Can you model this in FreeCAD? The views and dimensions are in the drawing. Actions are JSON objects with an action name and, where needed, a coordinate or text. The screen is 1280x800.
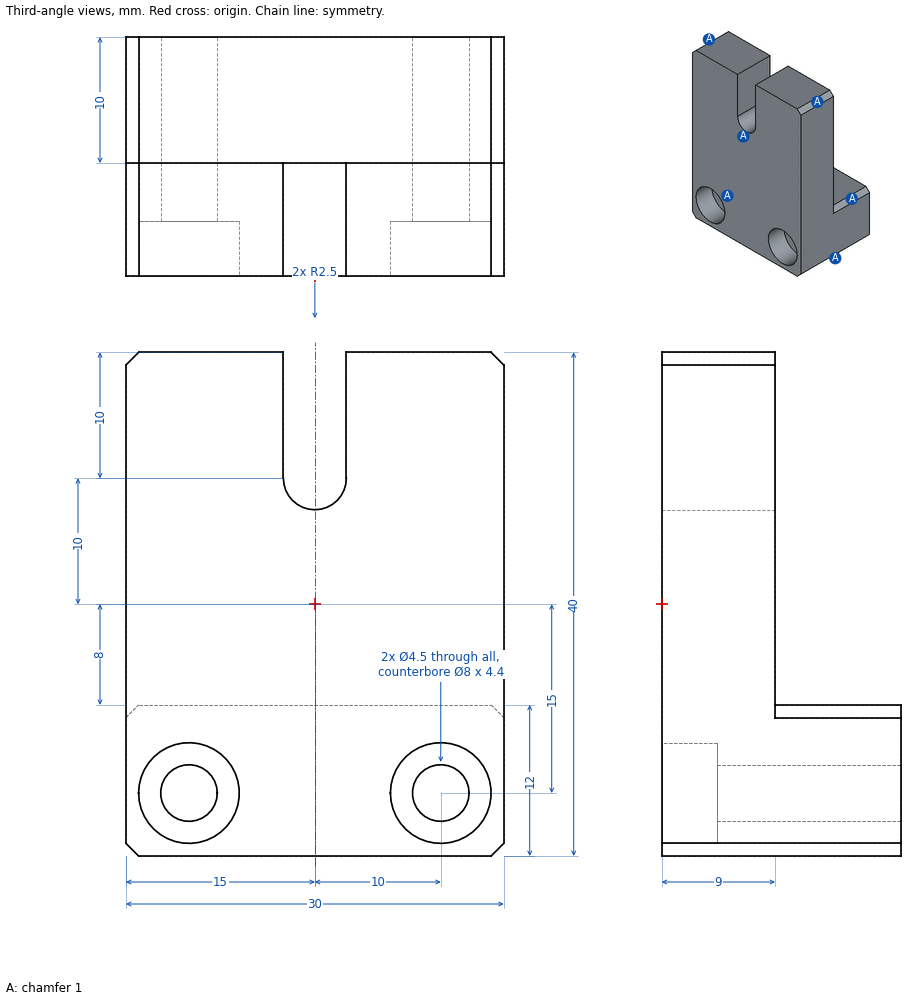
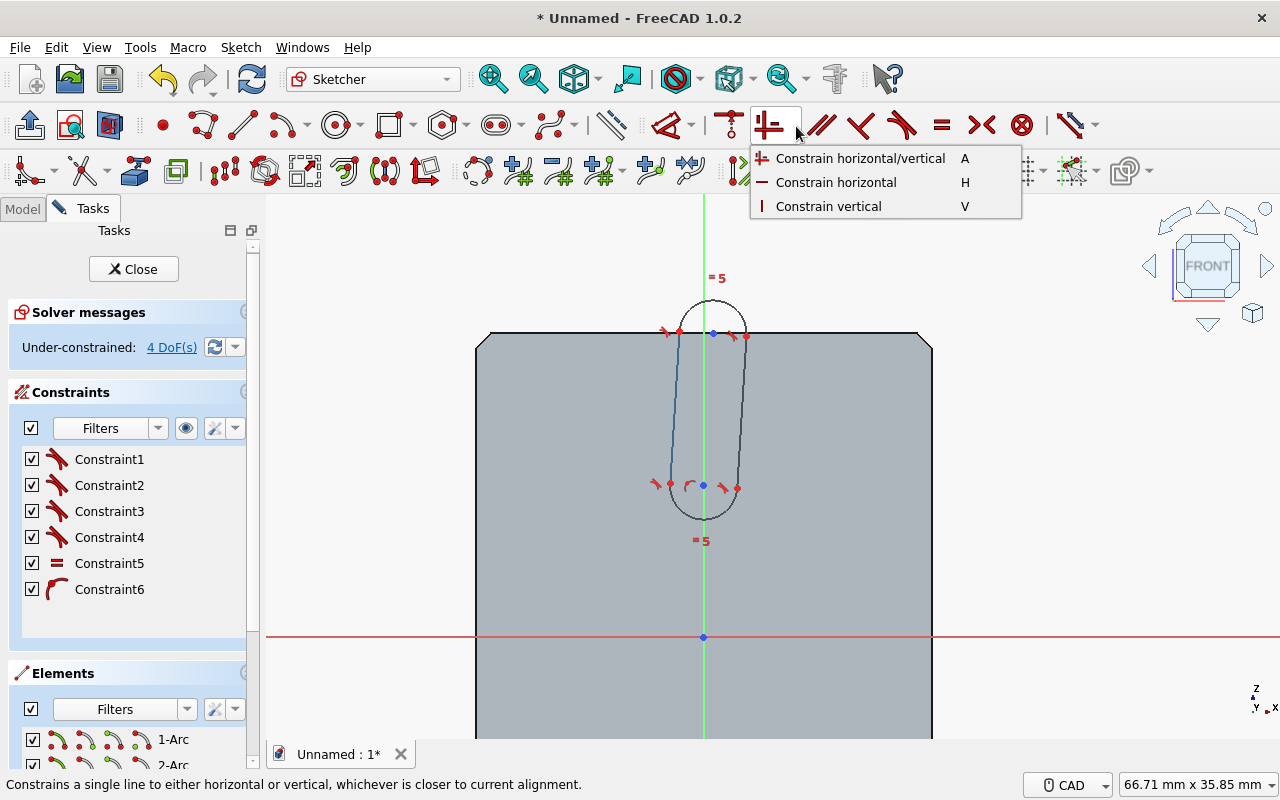
{"action": "left_click", "coordinate": [886, 206]}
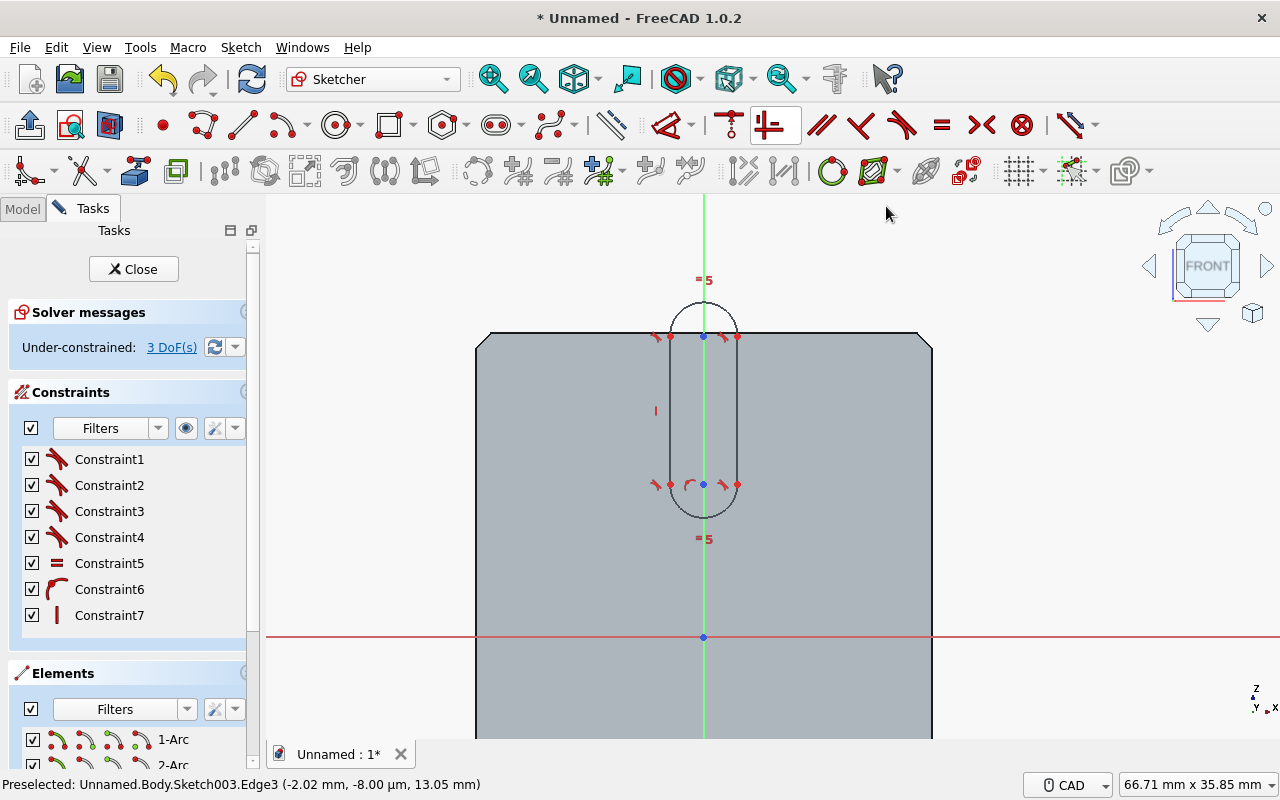
{"action": "left_click", "coordinate": [666, 126]}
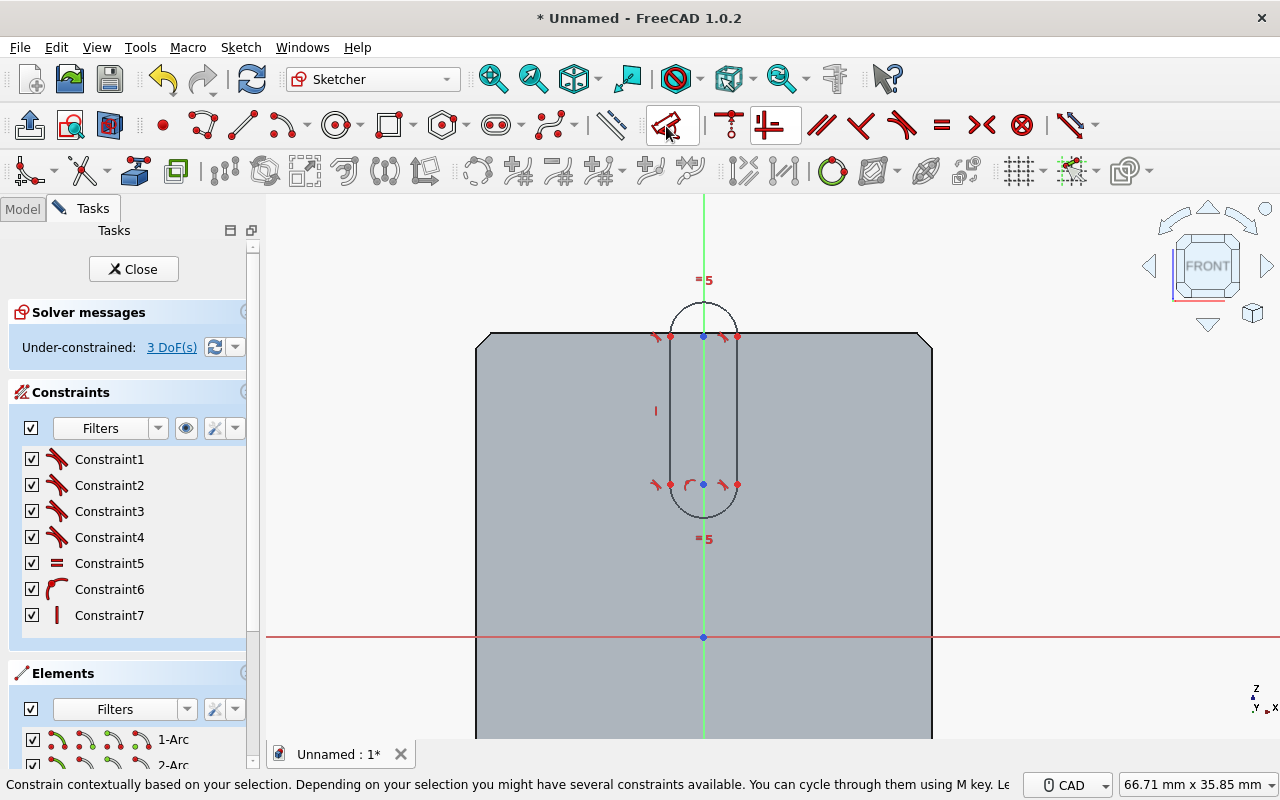
{"action": "left_click", "coordinate": [684, 511]}
{"action": "left_click", "coordinate": [665, 537]}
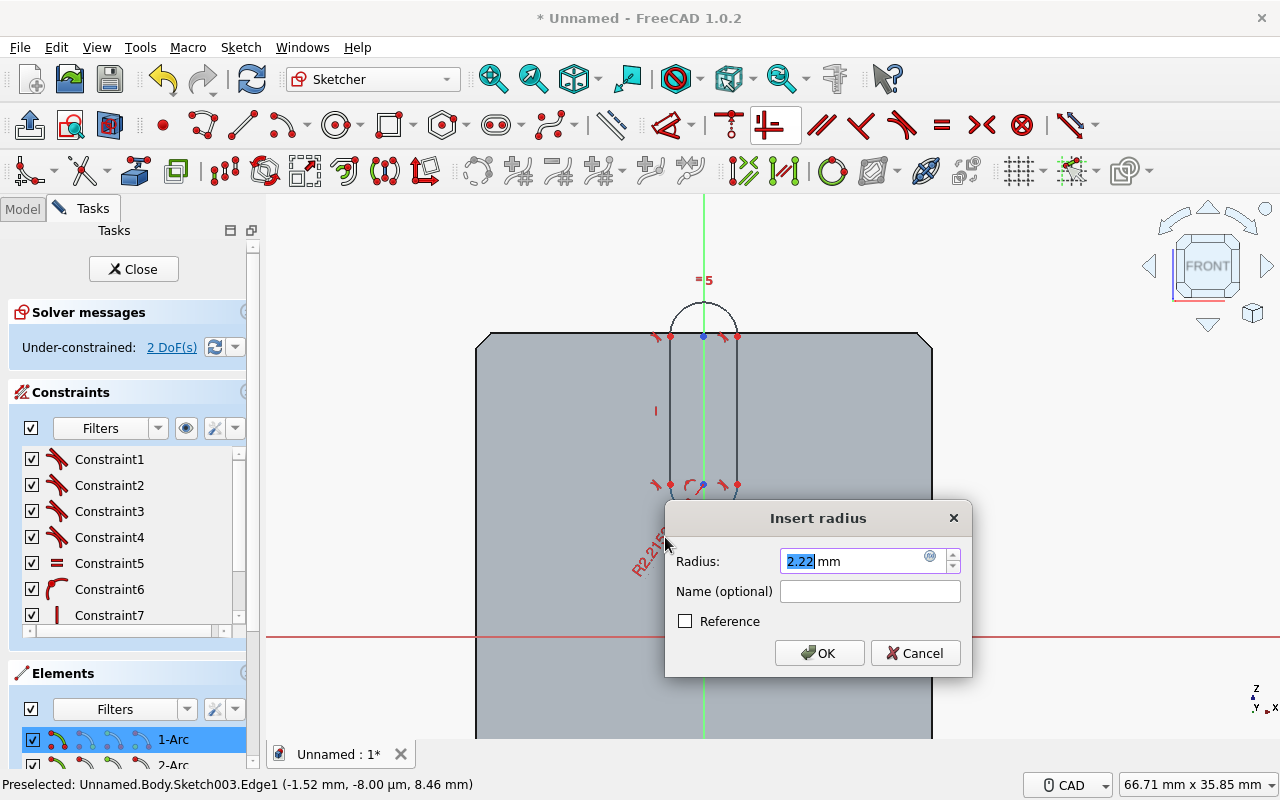
{"action": "type", "text": "2.5"}
{"action": "key", "text": "Return"}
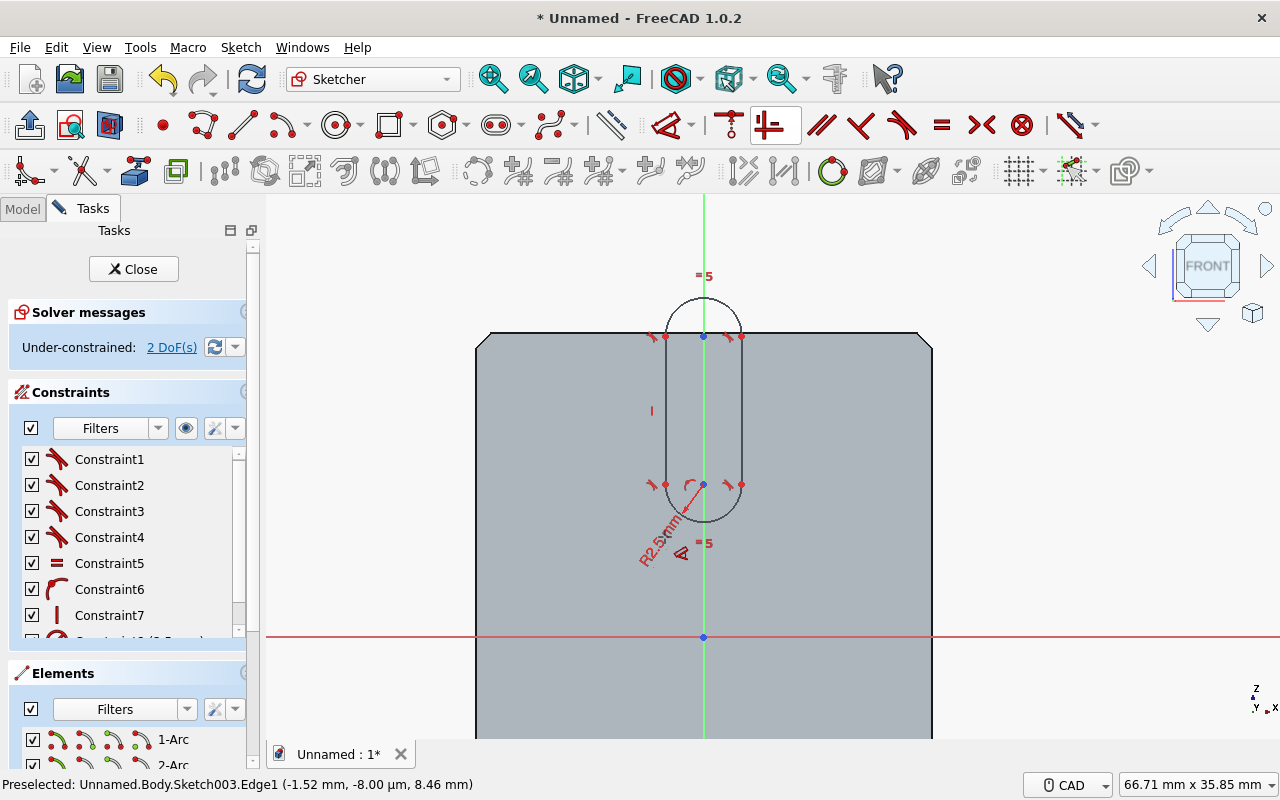
{"action": "left_click", "coordinate": [666, 440]}
{"action": "left_click", "coordinate": [632, 410]}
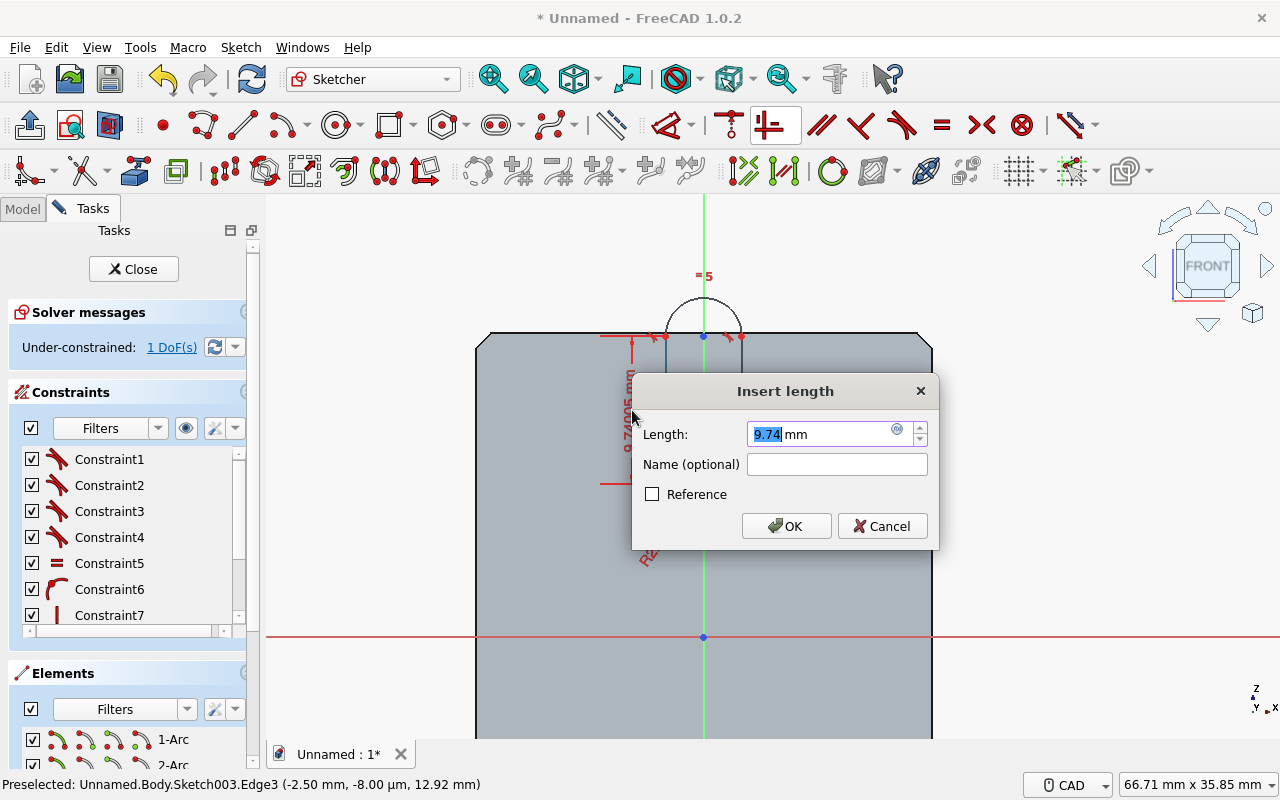
{"action": "type", "text": "10"}
{"action": "key", "text": "Return"}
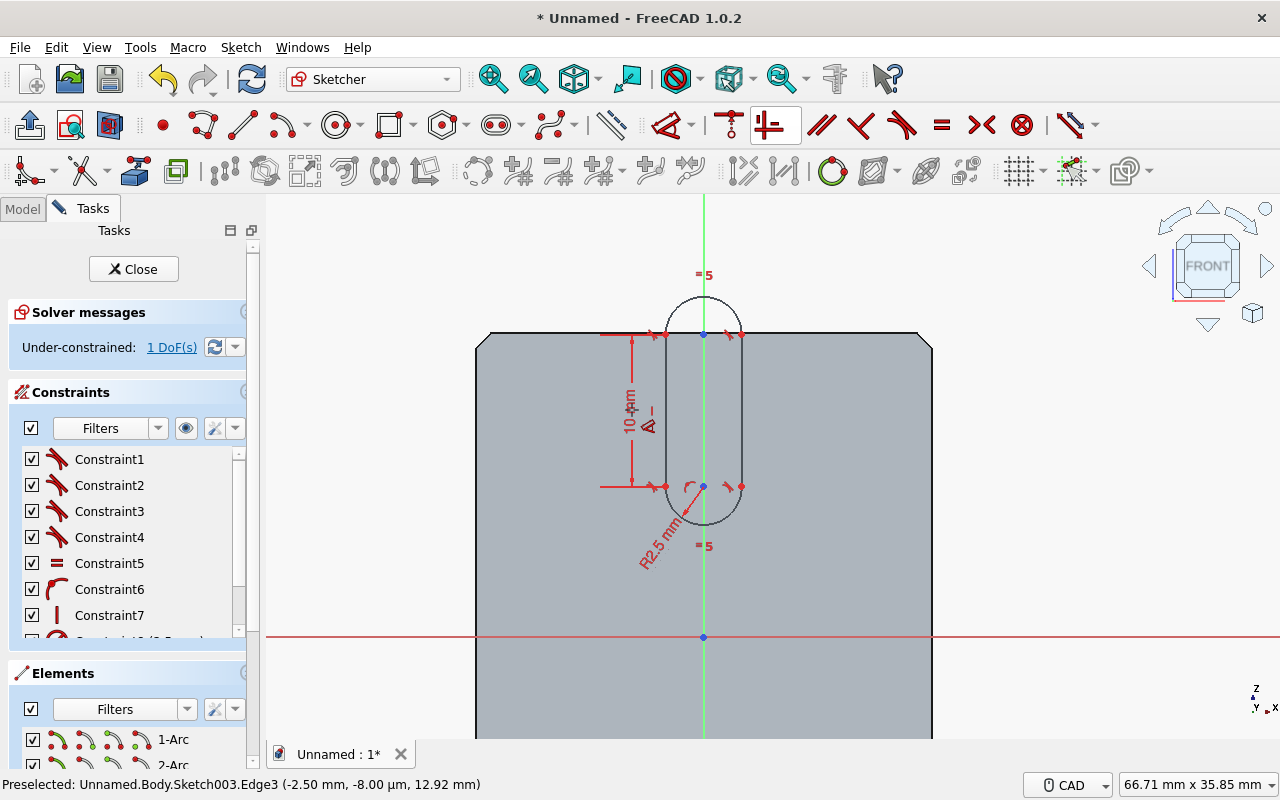
{"action": "left_click", "coordinate": [666, 487]}
{"action": "left_click", "coordinate": [632, 562]}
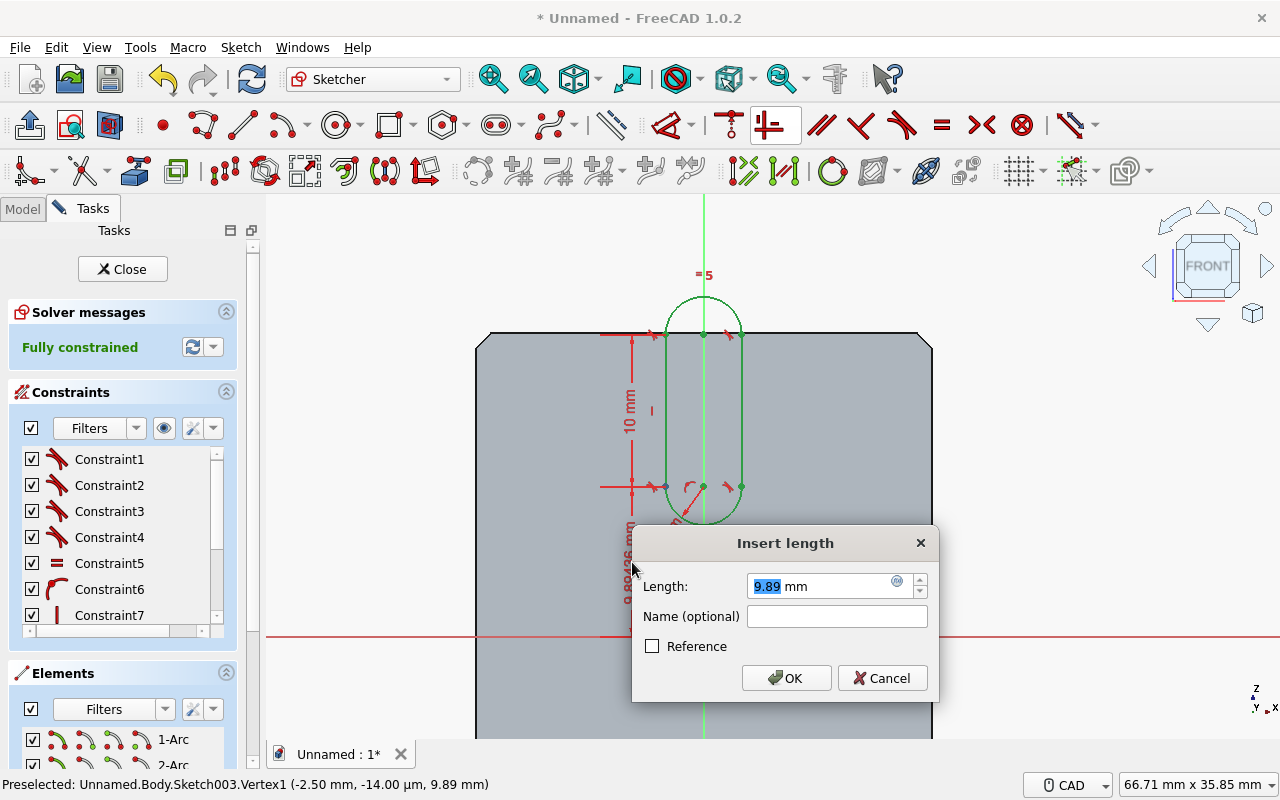
{"action": "type", "text": "10"}
{"action": "key", "text": "Return"}
{"action": "key", "text": "Escape"}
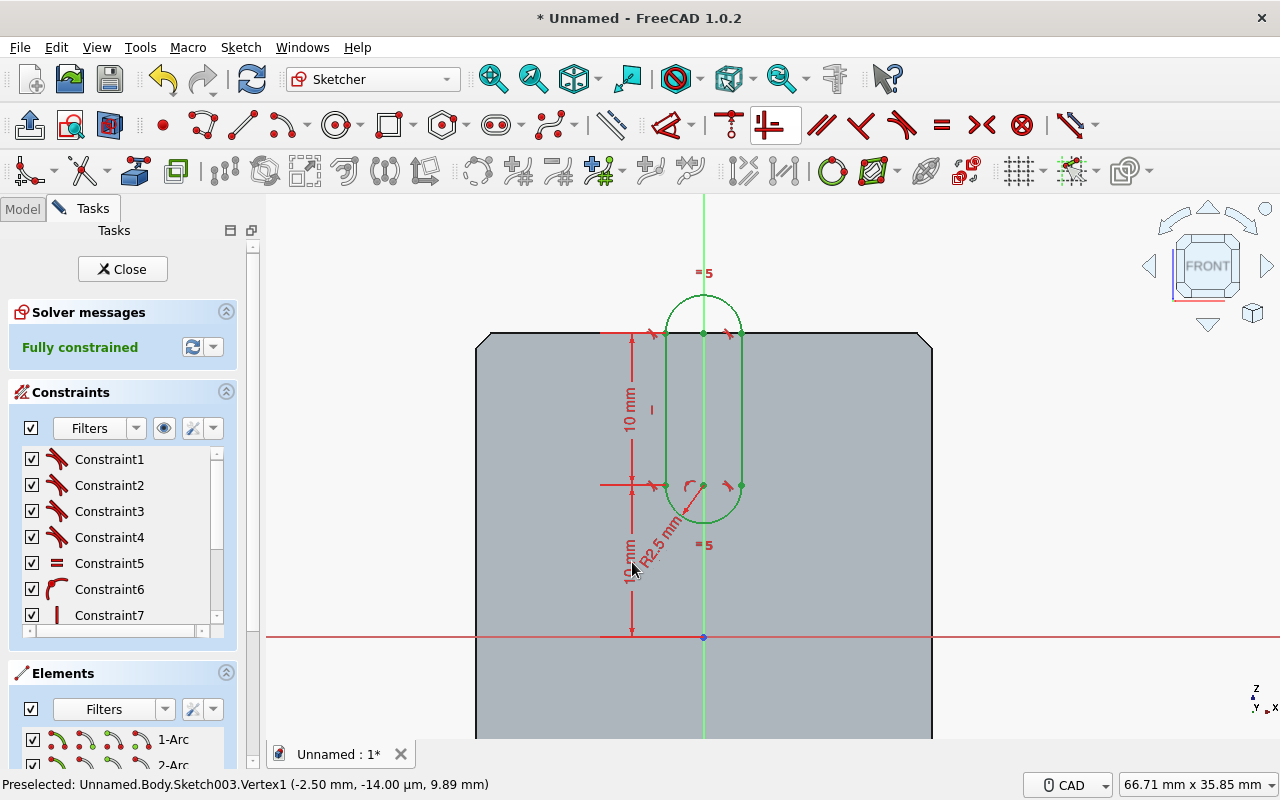
{"action": "left_click", "coordinate": [123, 269]}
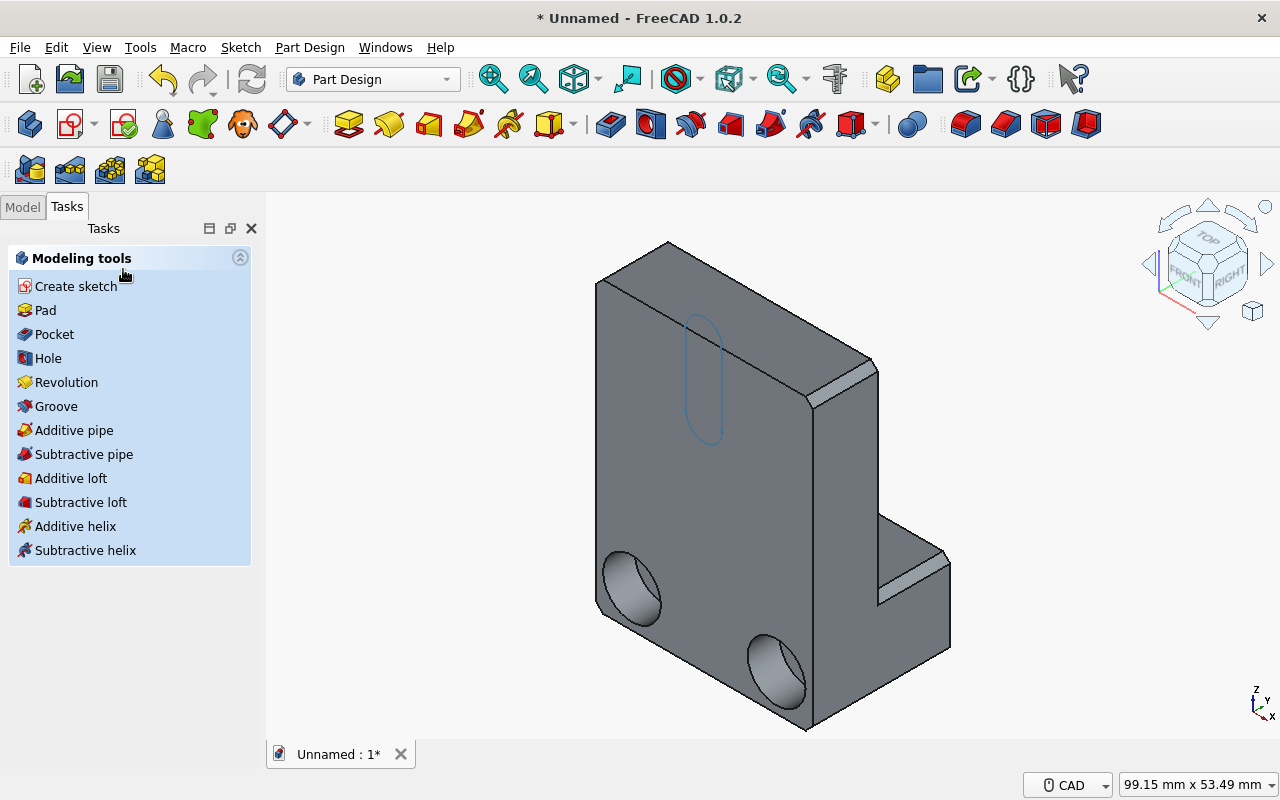
{"action": "left_click", "coordinate": [612, 124]}